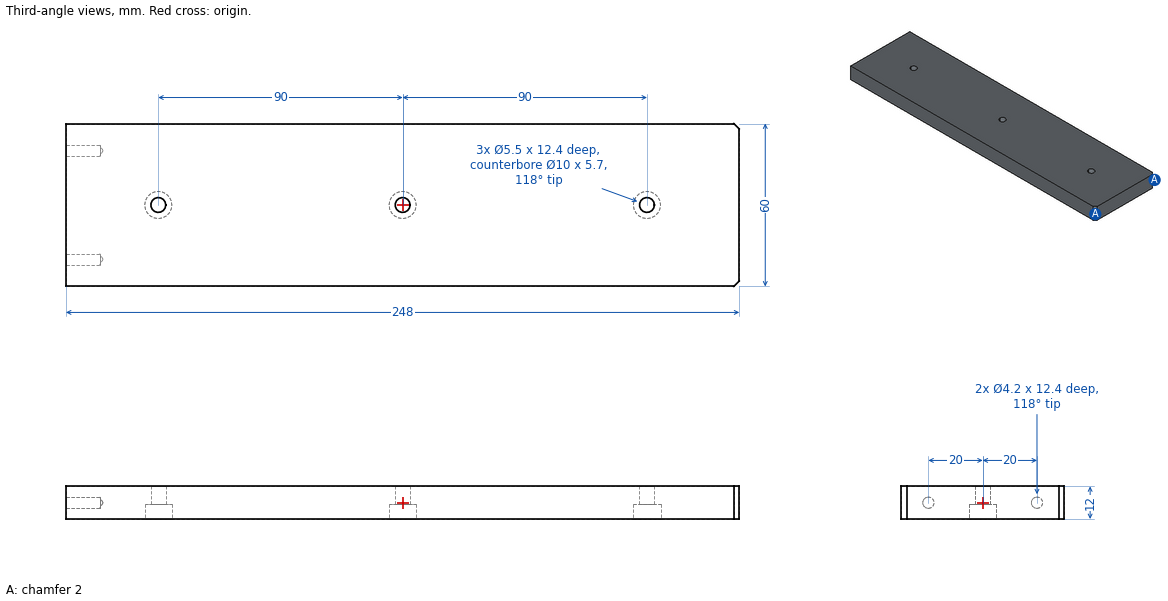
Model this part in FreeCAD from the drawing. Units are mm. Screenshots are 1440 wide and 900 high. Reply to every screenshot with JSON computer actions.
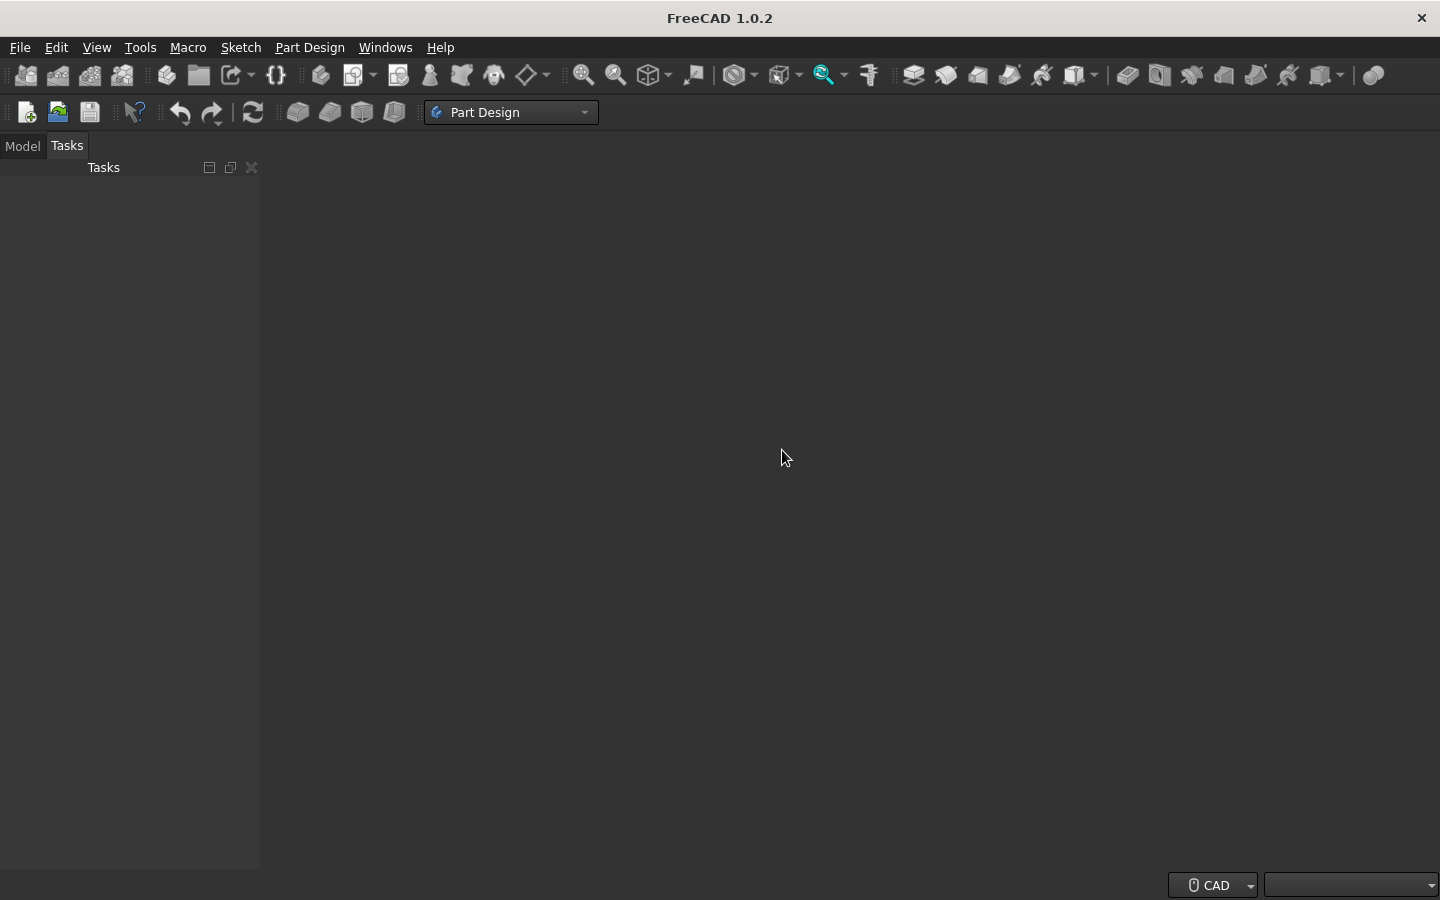
{"action": "left_click", "coordinate": [26, 112]}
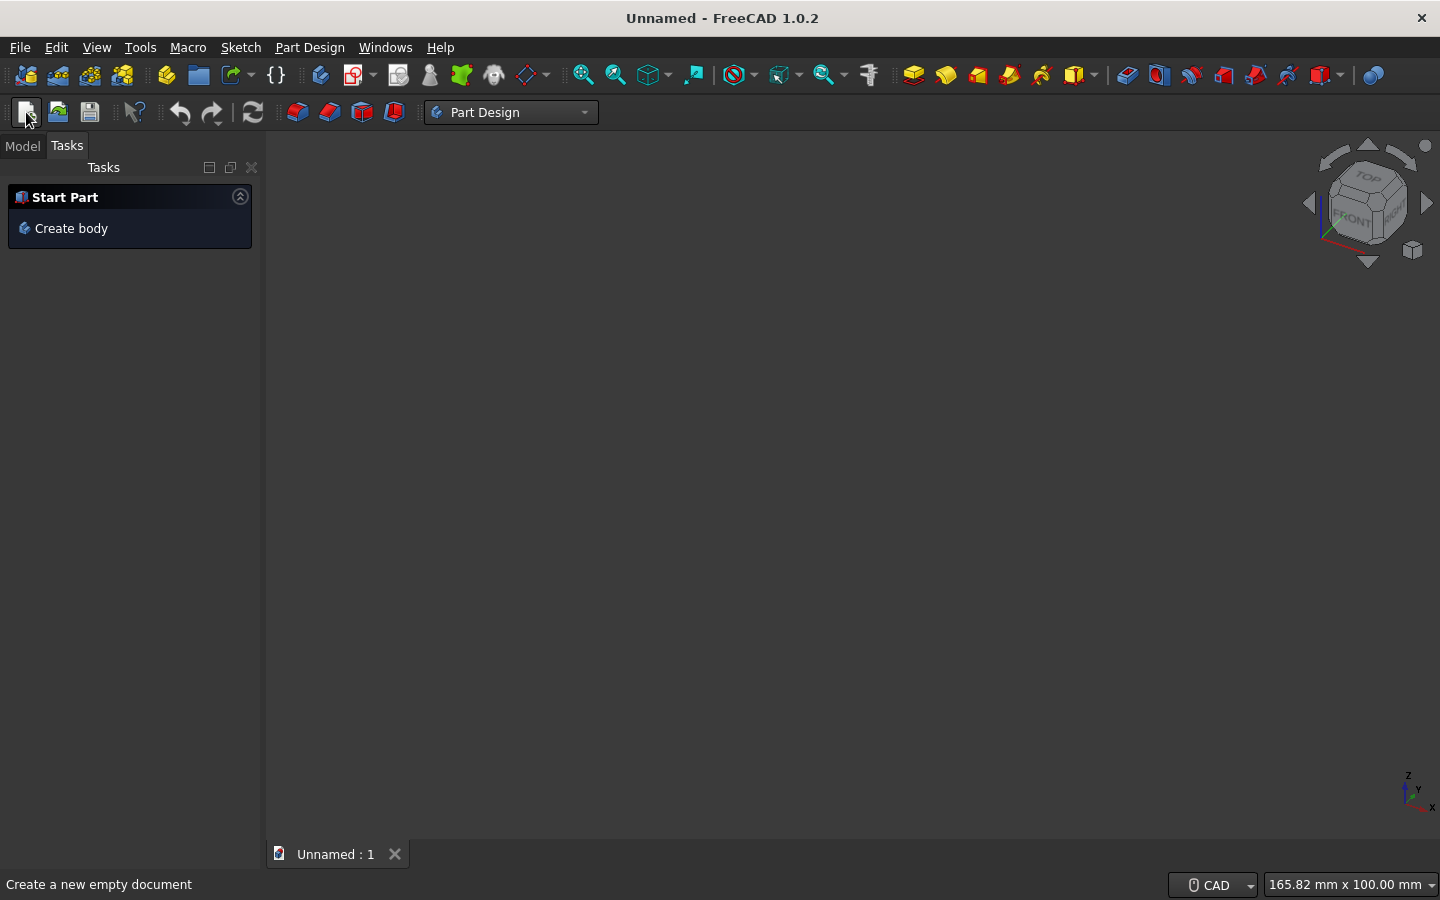
{"action": "left_click", "coordinate": [354, 76]}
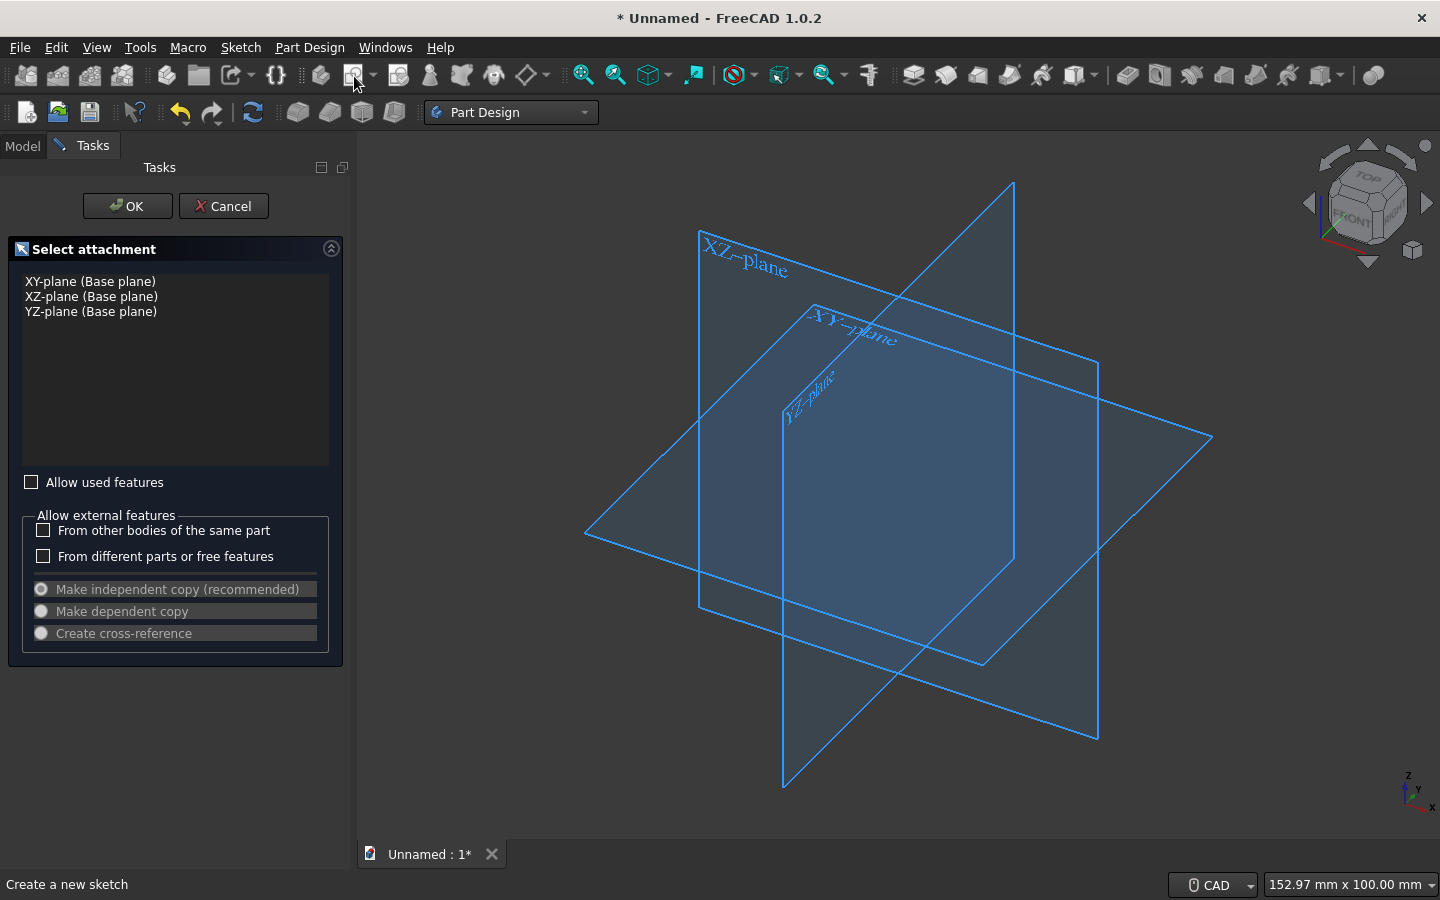
{"action": "left_click", "coordinate": [82, 282]}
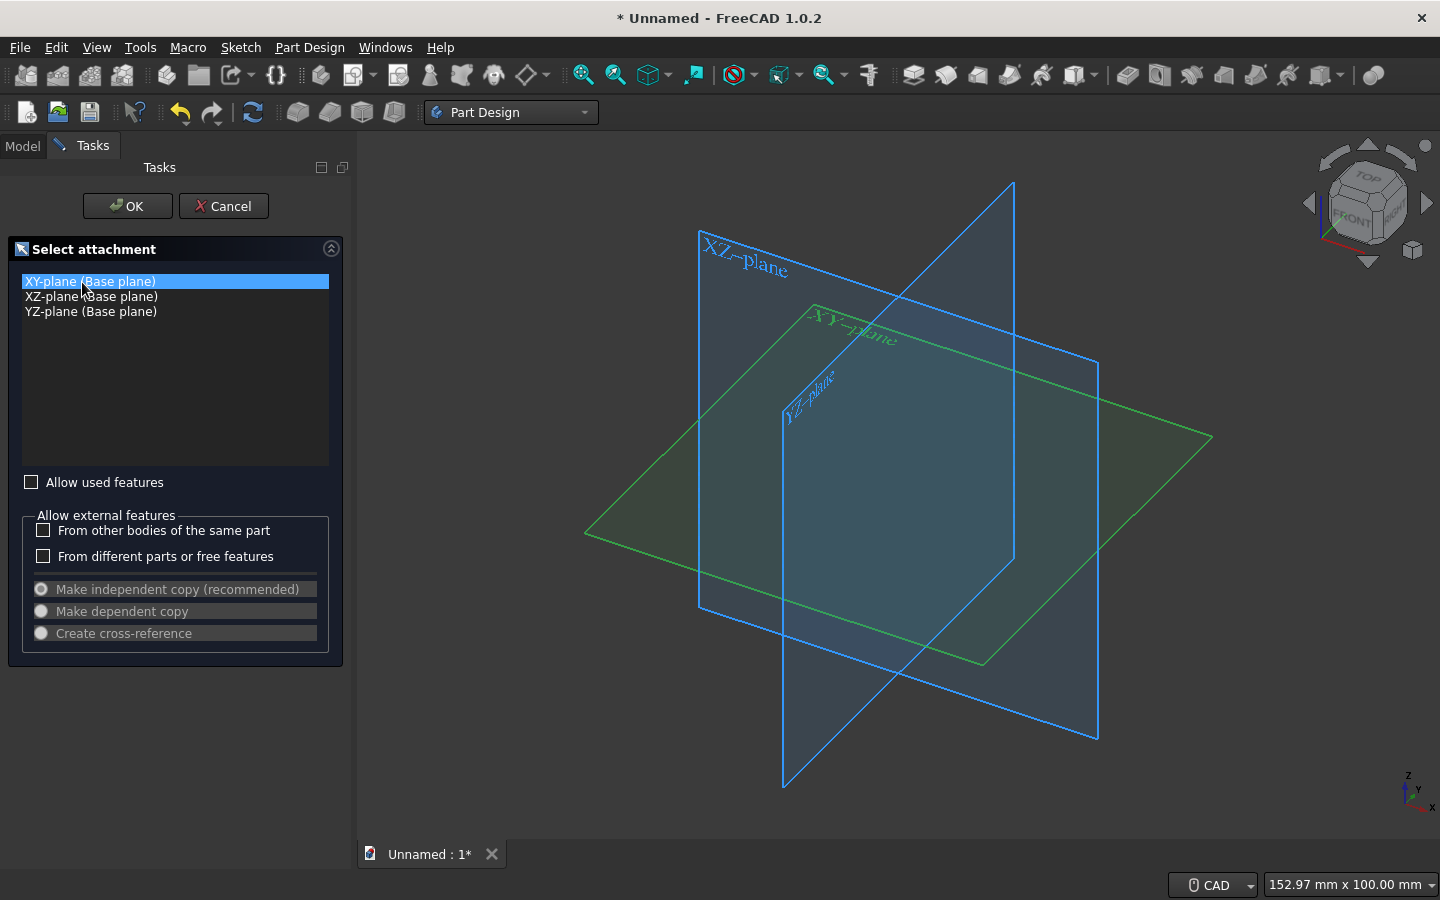
{"action": "left_click", "coordinate": [128, 206]}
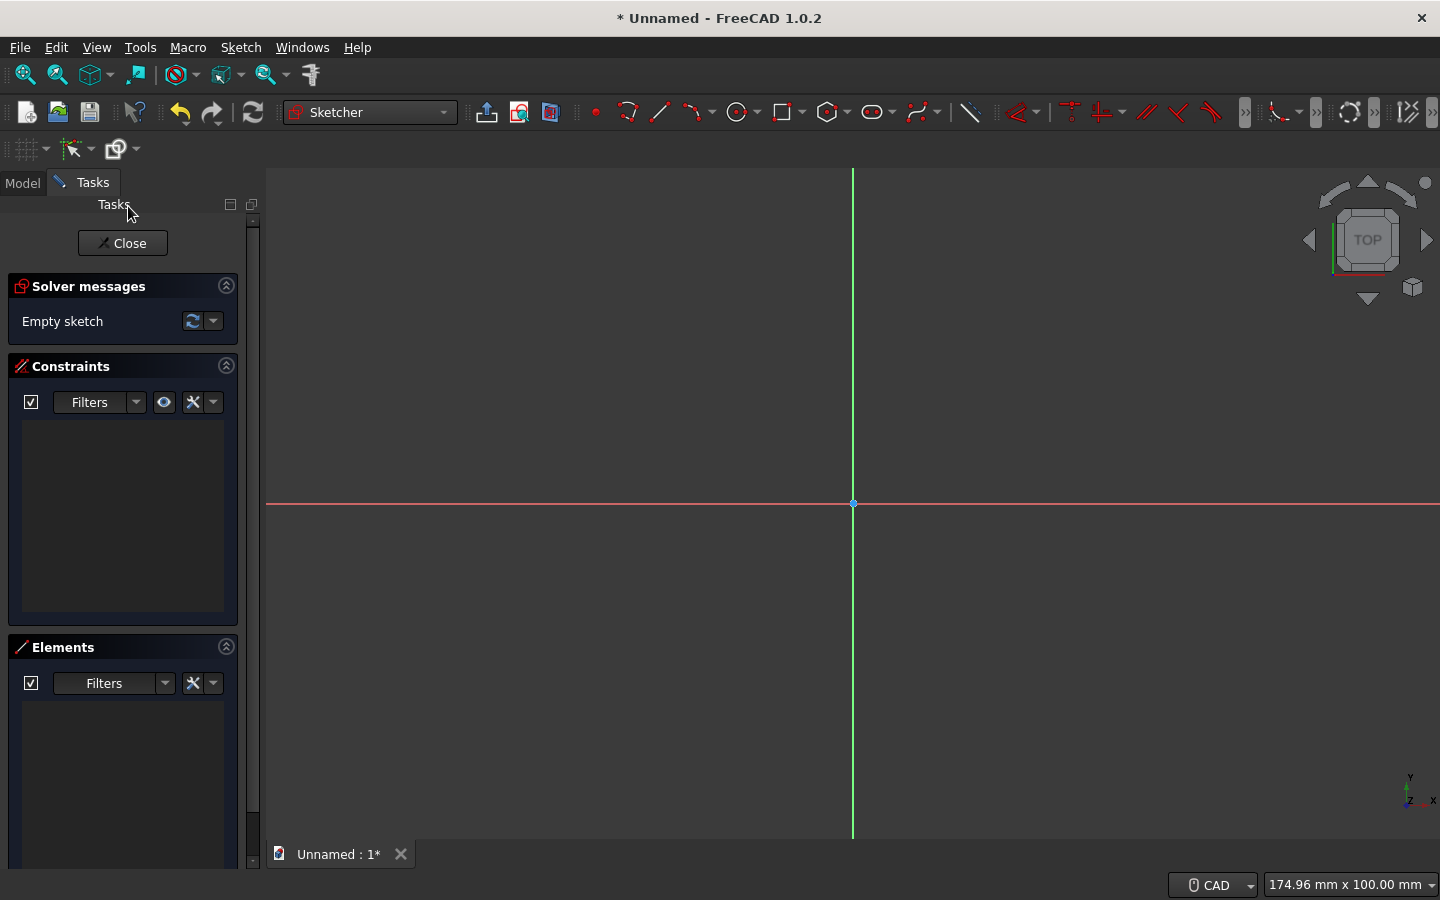
{"action": "scroll", "coordinate": [729, 503], "scroll_direction": "down", "scroll_amount": 4}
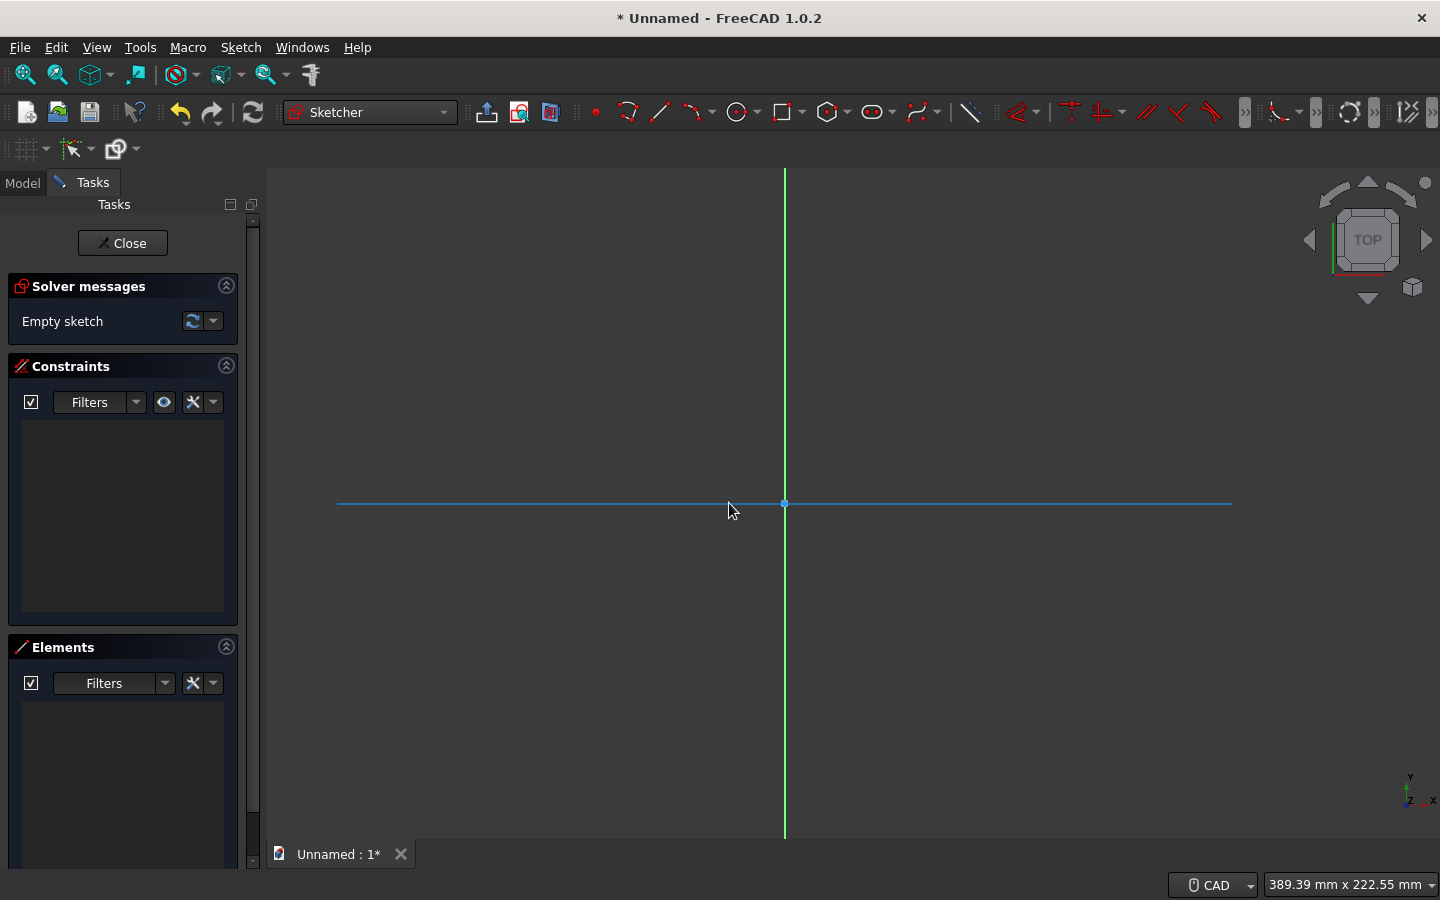
{"action": "key", "text": "g v"}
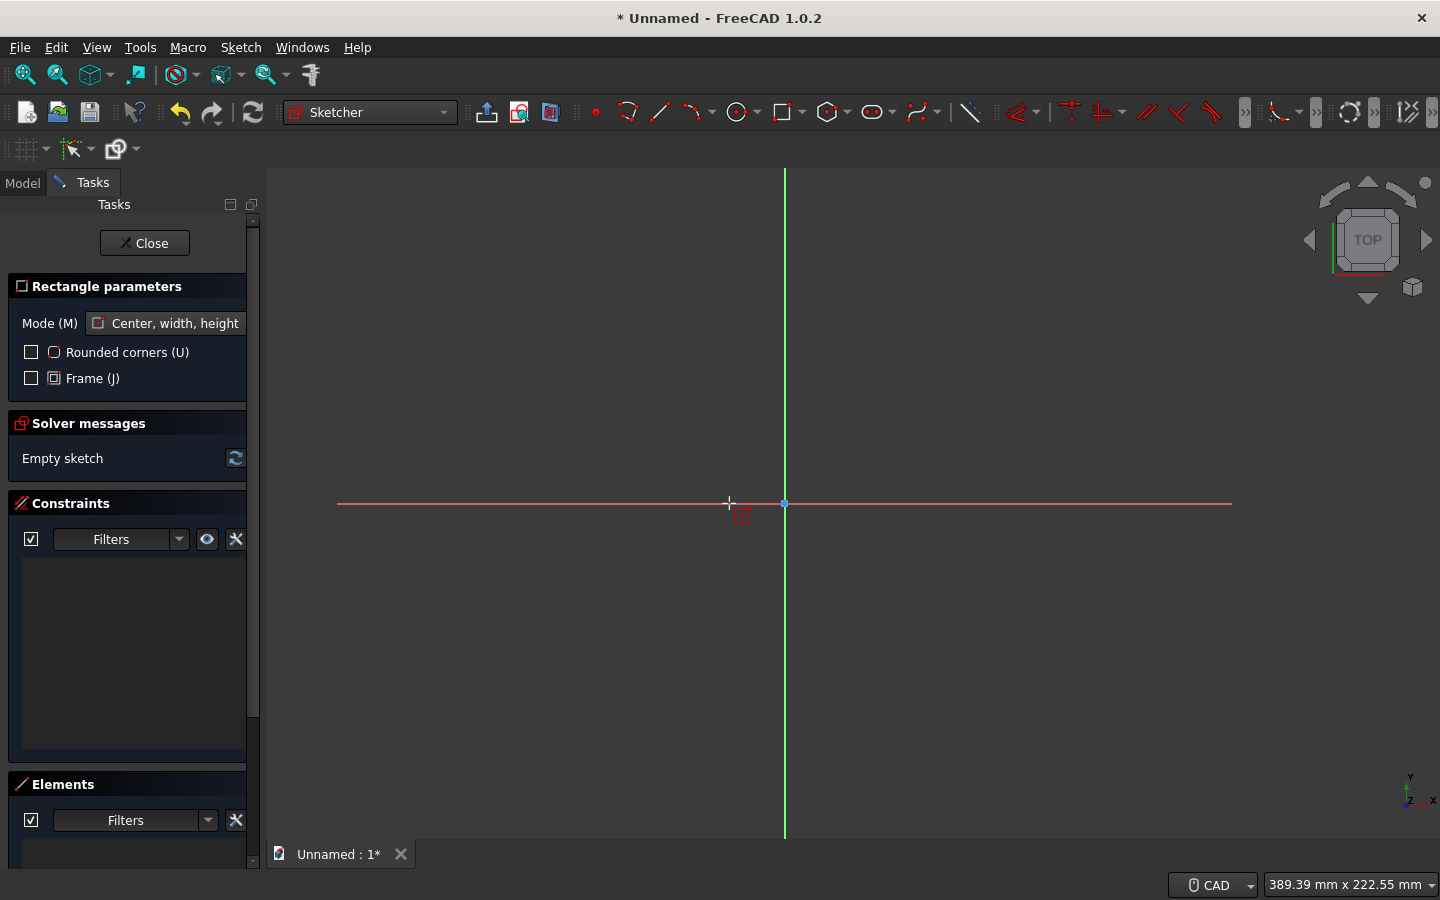
{"action": "left_click", "coordinate": [785, 504]}
{"action": "left_click", "coordinate": [1159, 413]}
{"action": "key", "text": "Escape"}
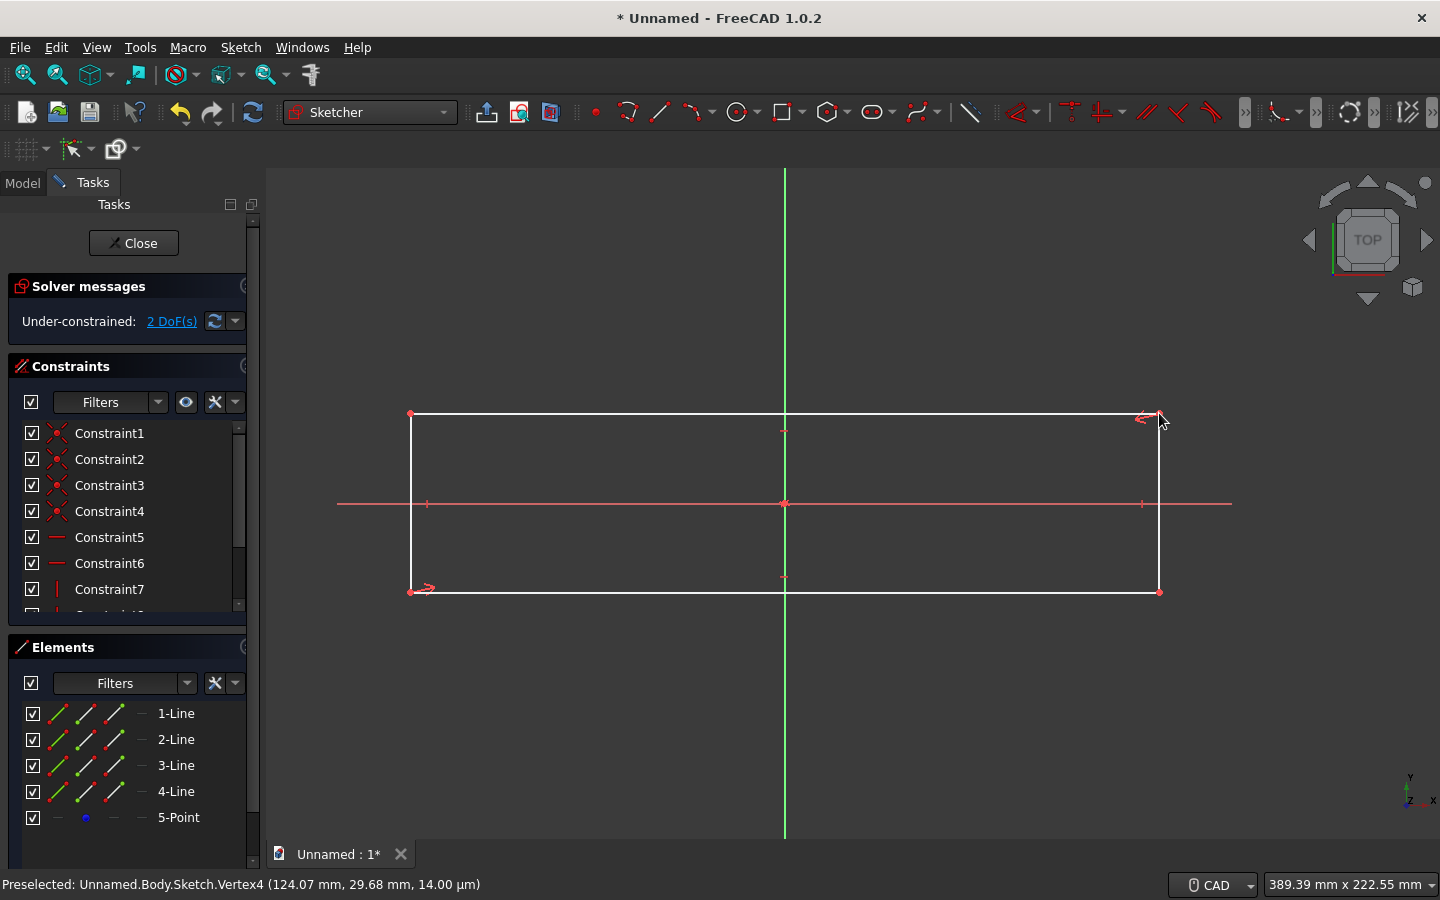
{"action": "left_click", "coordinate": [1016, 112]}